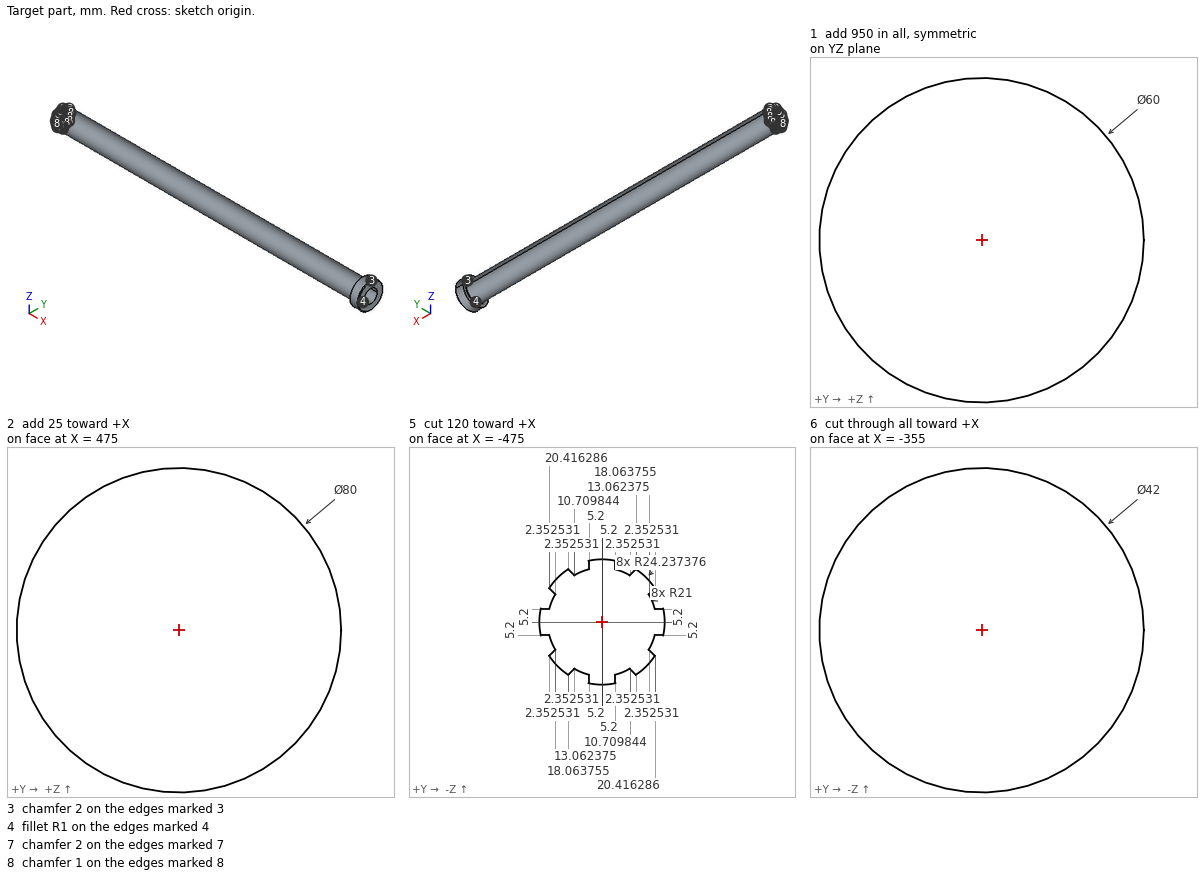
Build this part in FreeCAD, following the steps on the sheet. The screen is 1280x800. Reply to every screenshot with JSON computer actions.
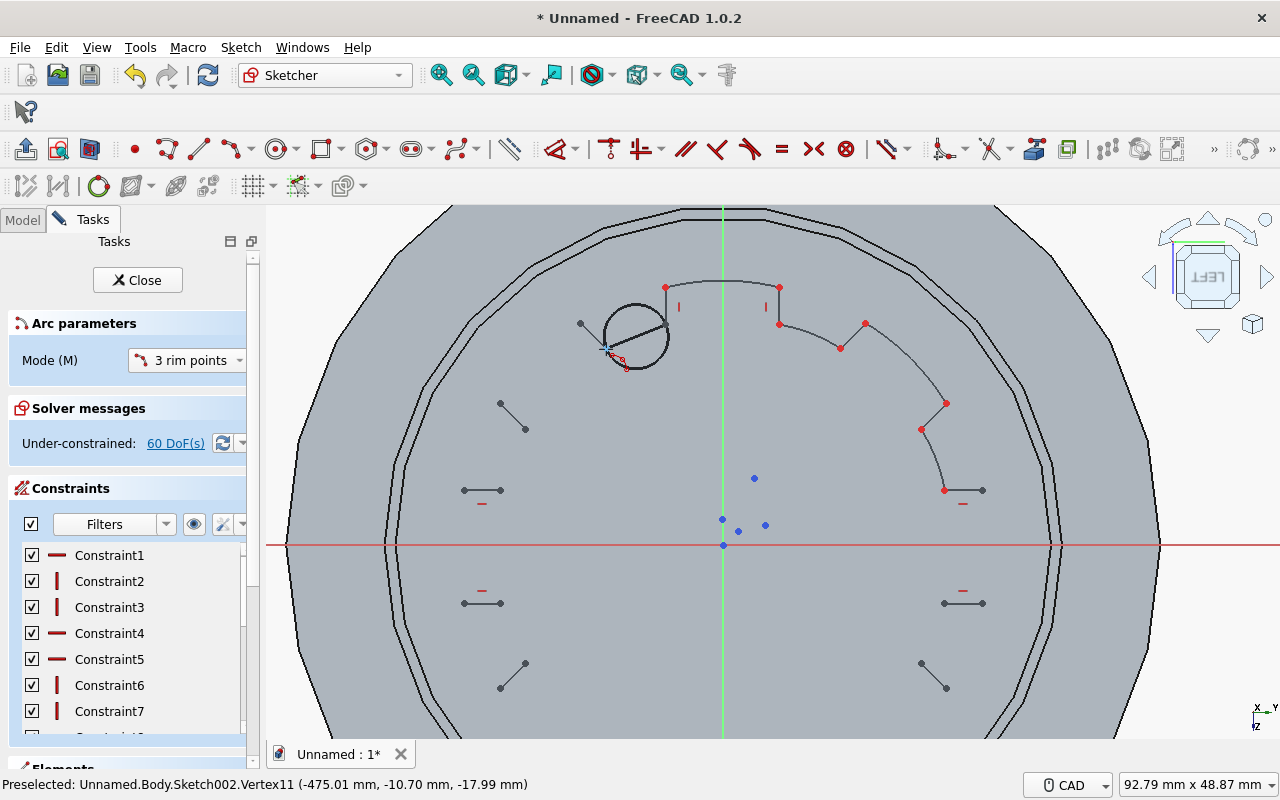
{"action": "scroll", "coordinate": [635, 333], "scroll_direction": "up", "scroll_amount": 10}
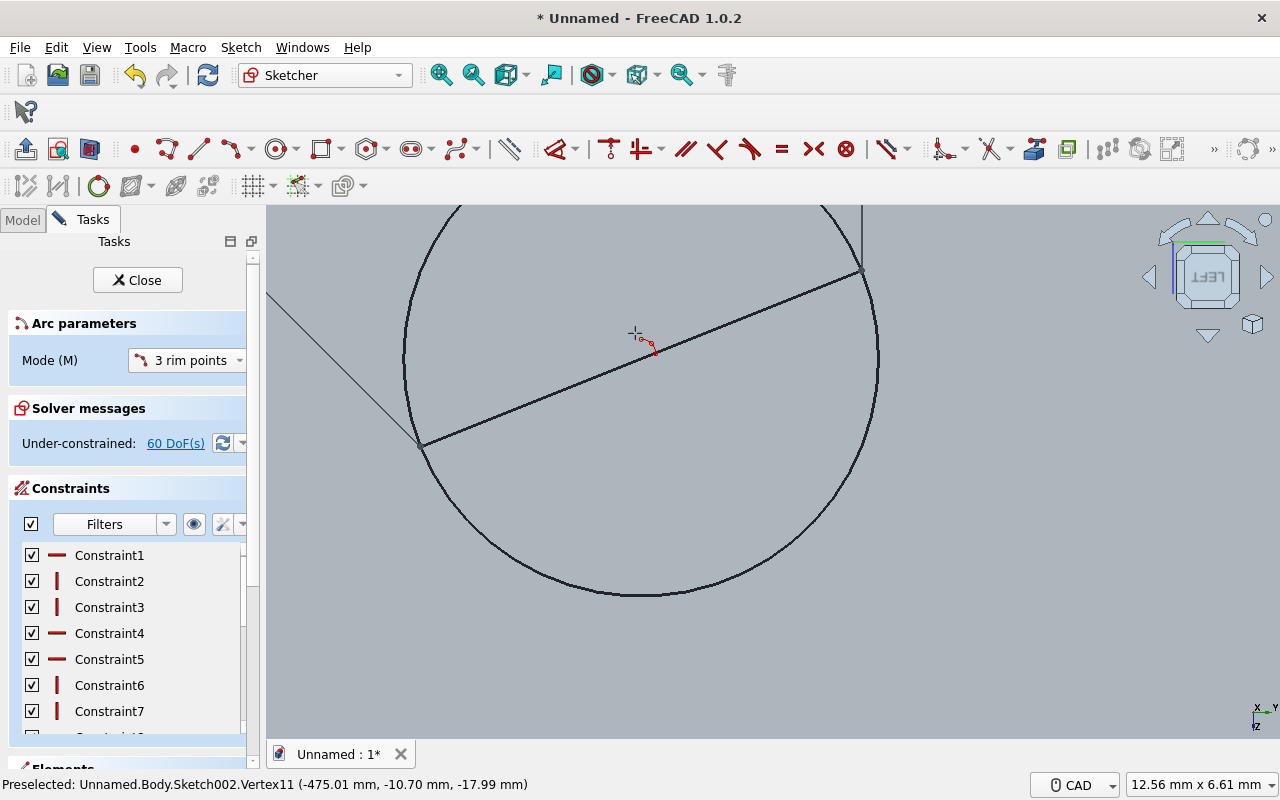
{"action": "left_click", "coordinate": [636, 333]}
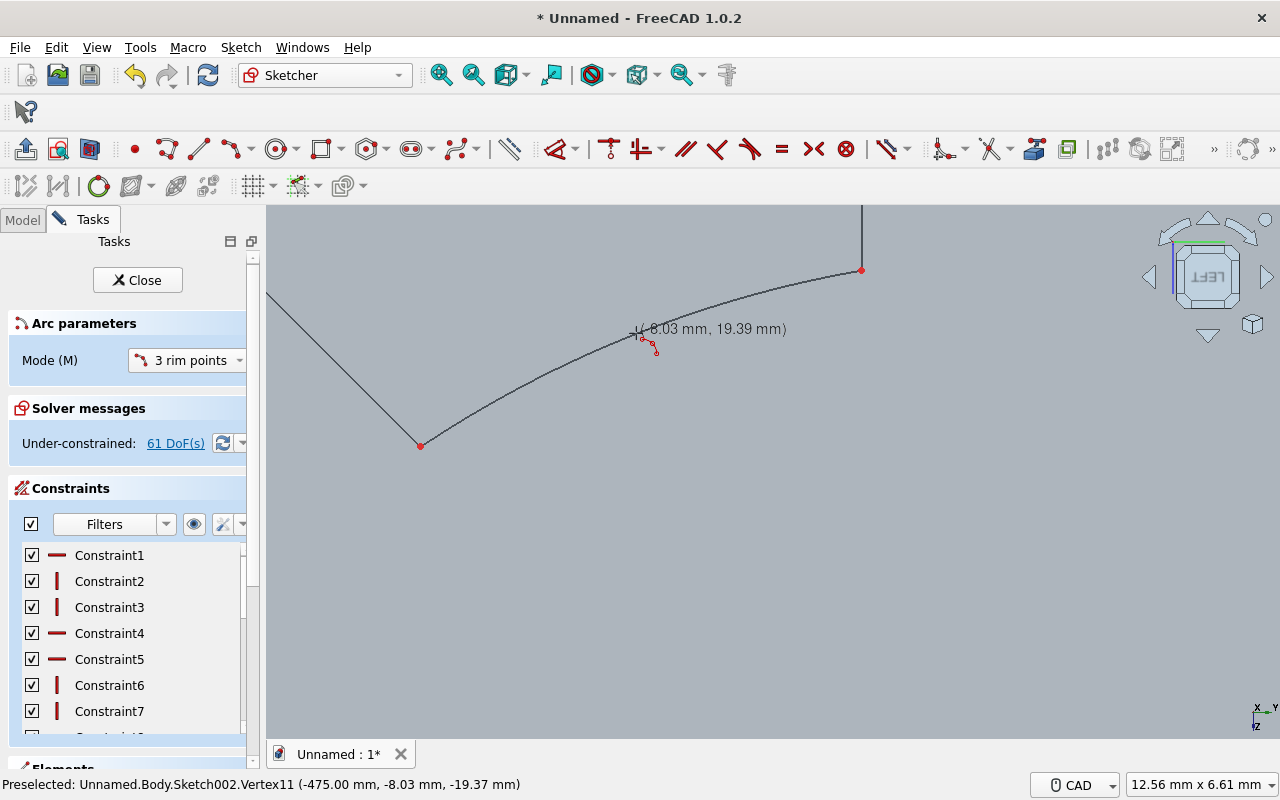
{"action": "scroll", "coordinate": [647, 330], "scroll_direction": "down", "scroll_amount": 12}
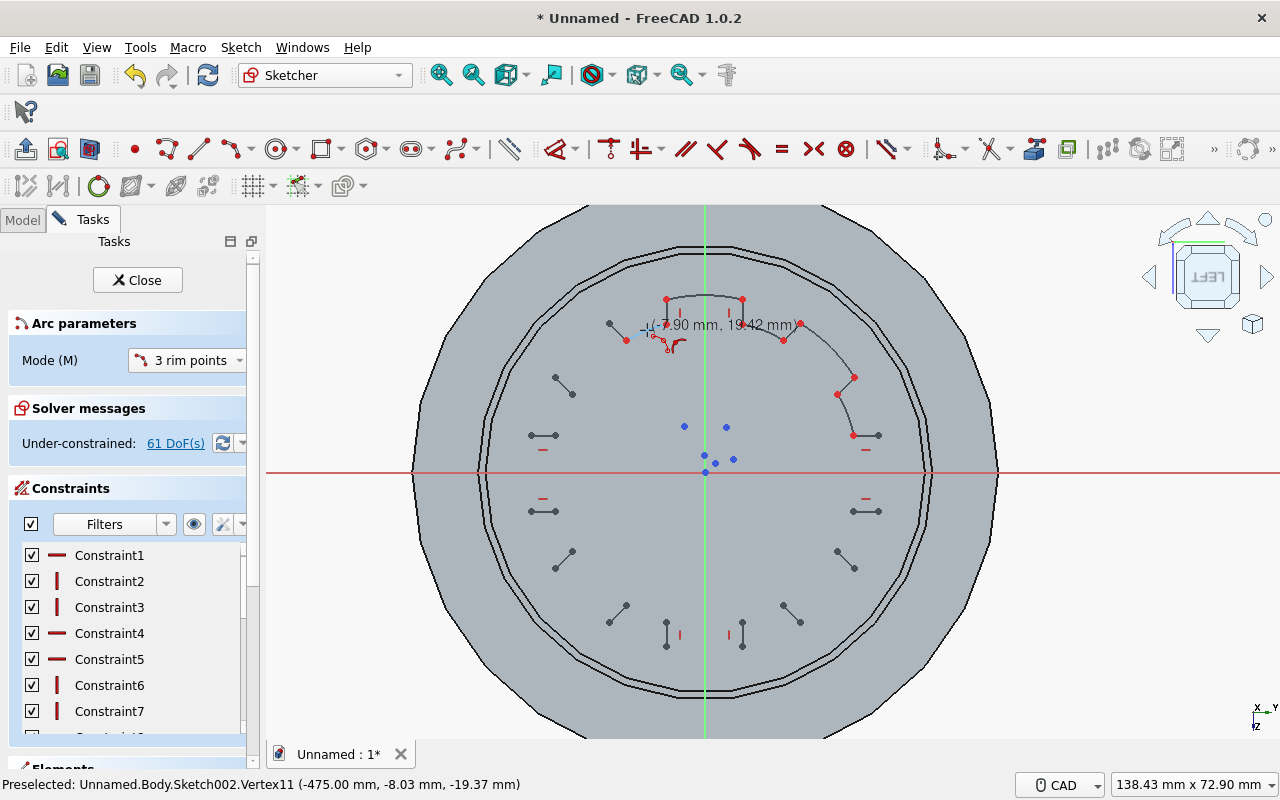
{"action": "scroll", "coordinate": [610, 323], "scroll_direction": "up", "scroll_amount": 2}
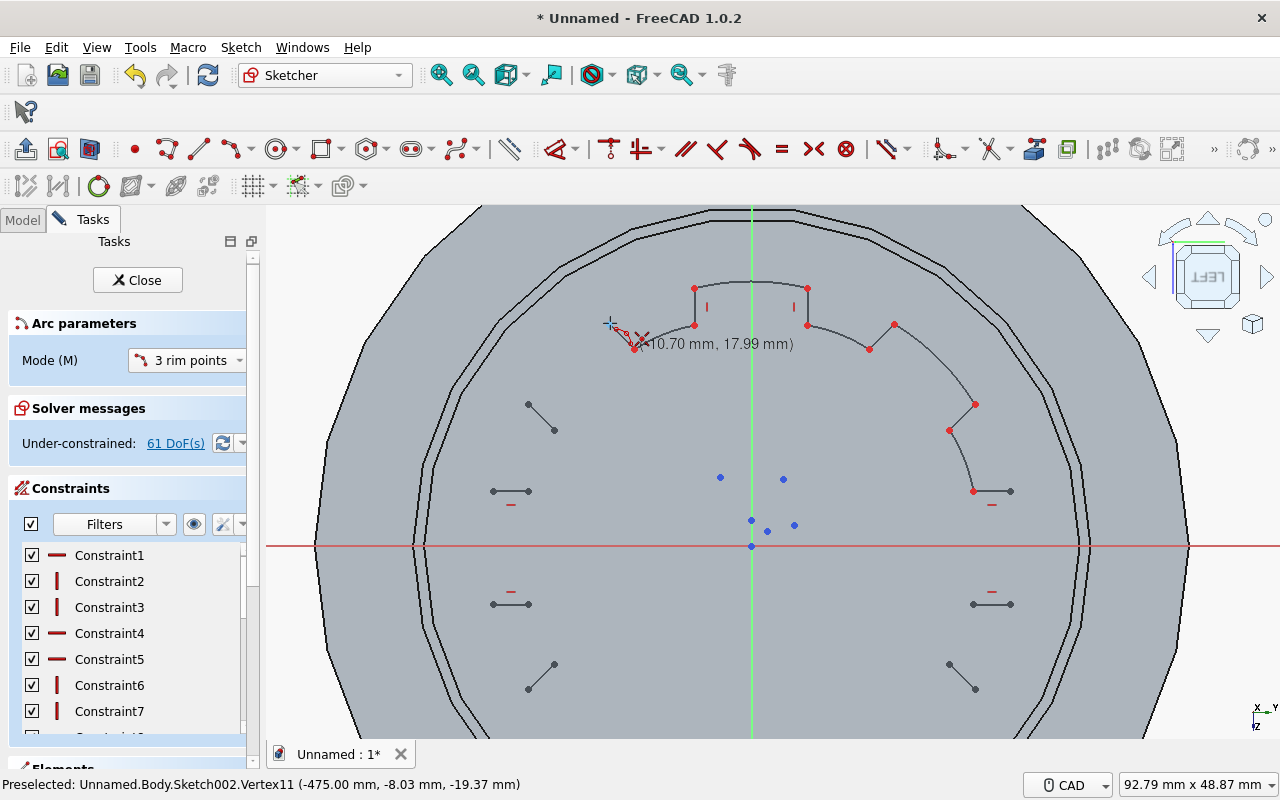
{"action": "left_click", "coordinate": [610, 324]}
{"action": "left_click", "coordinate": [529, 405]}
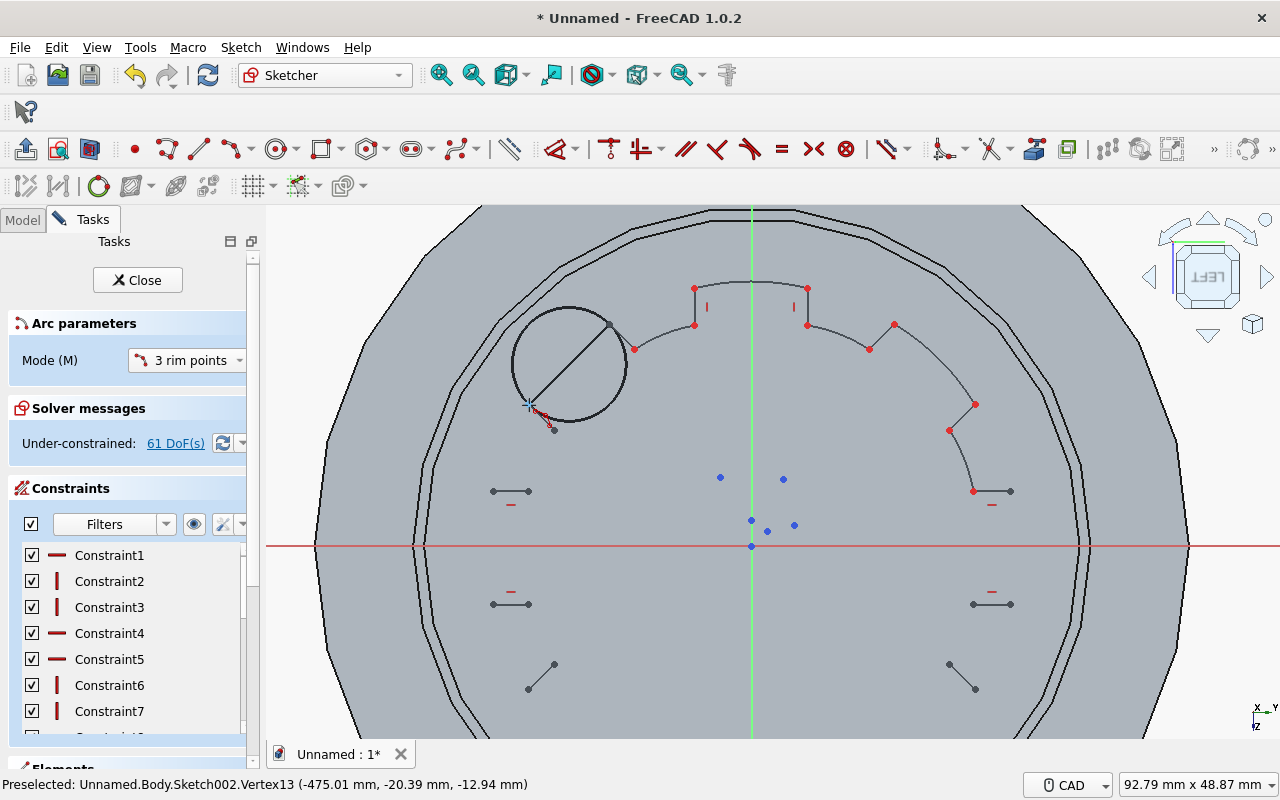
{"action": "scroll", "coordinate": [565, 359], "scroll_direction": "up", "scroll_amount": 5}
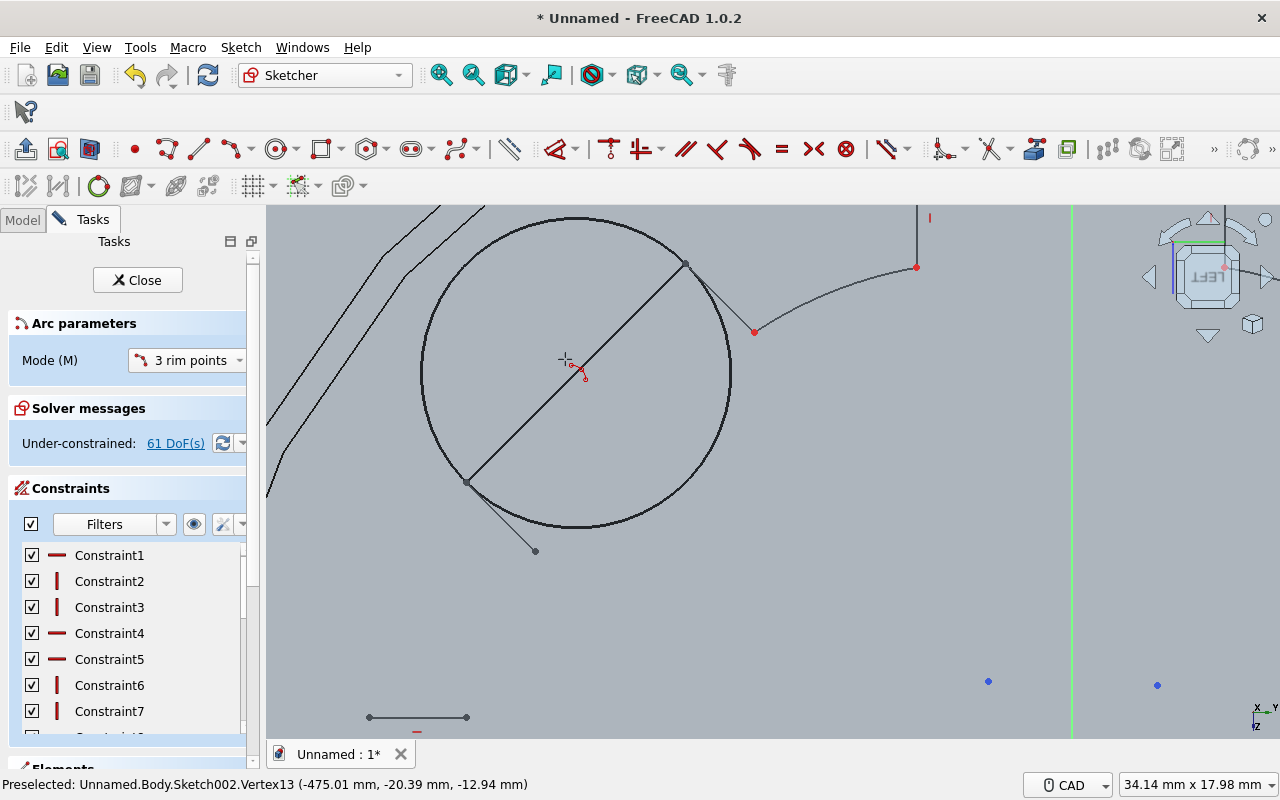
{"action": "left_click", "coordinate": [563, 358]}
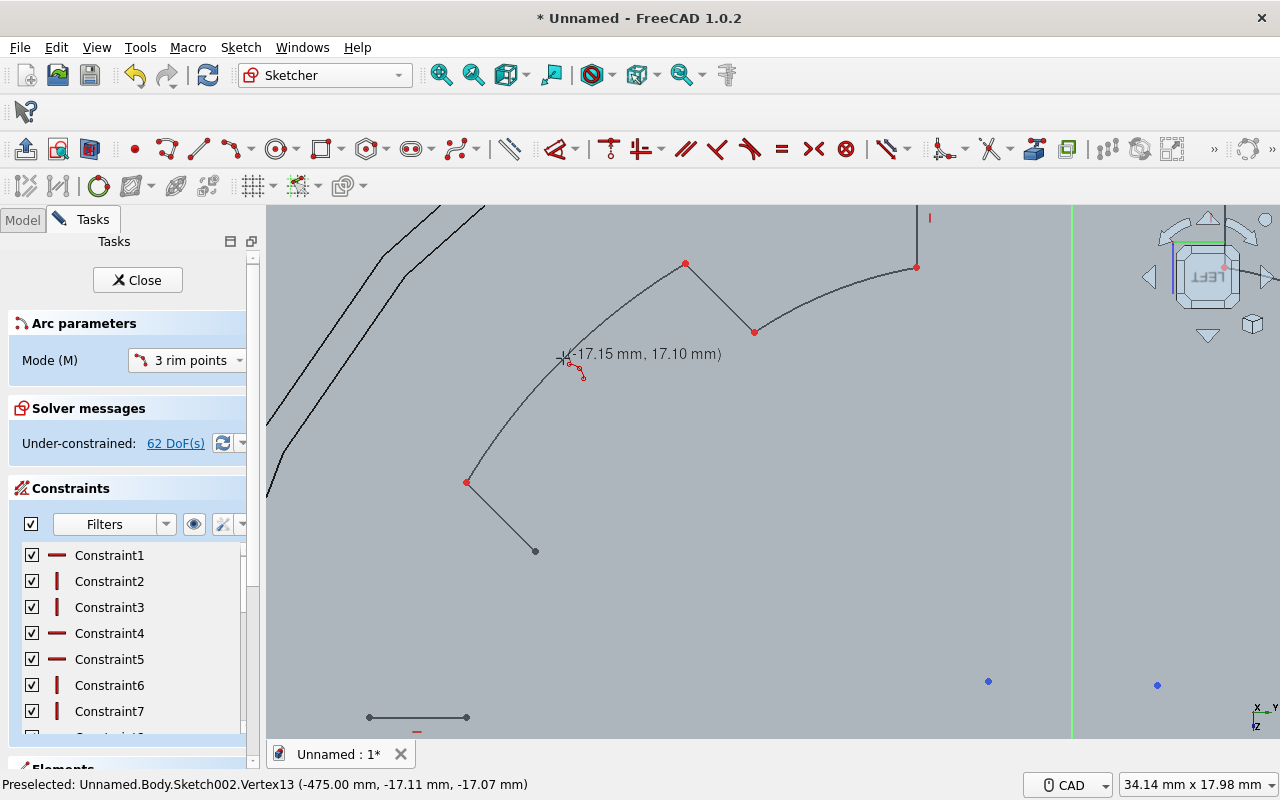
{"action": "scroll", "coordinate": [584, 343], "scroll_direction": "down", "scroll_amount": 7}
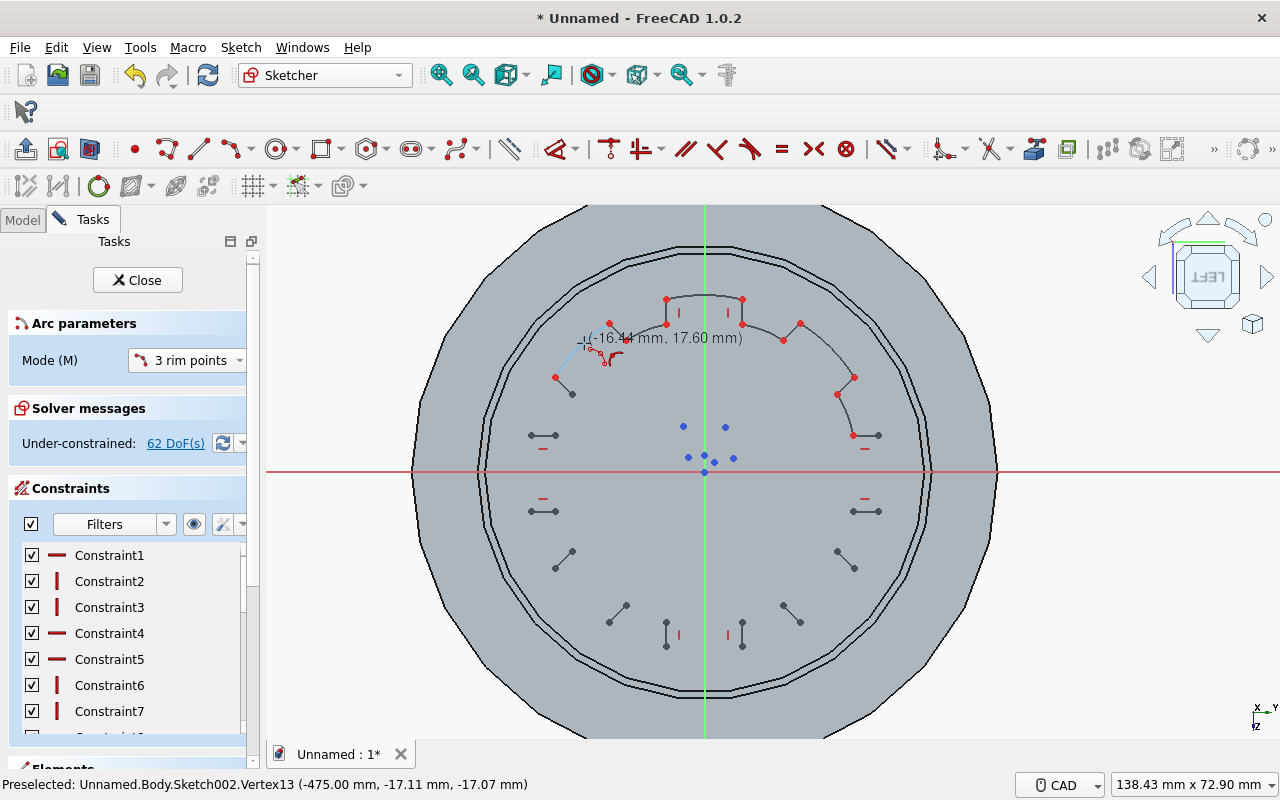
{"action": "scroll", "coordinate": [572, 394], "scroll_direction": "up", "scroll_amount": 2}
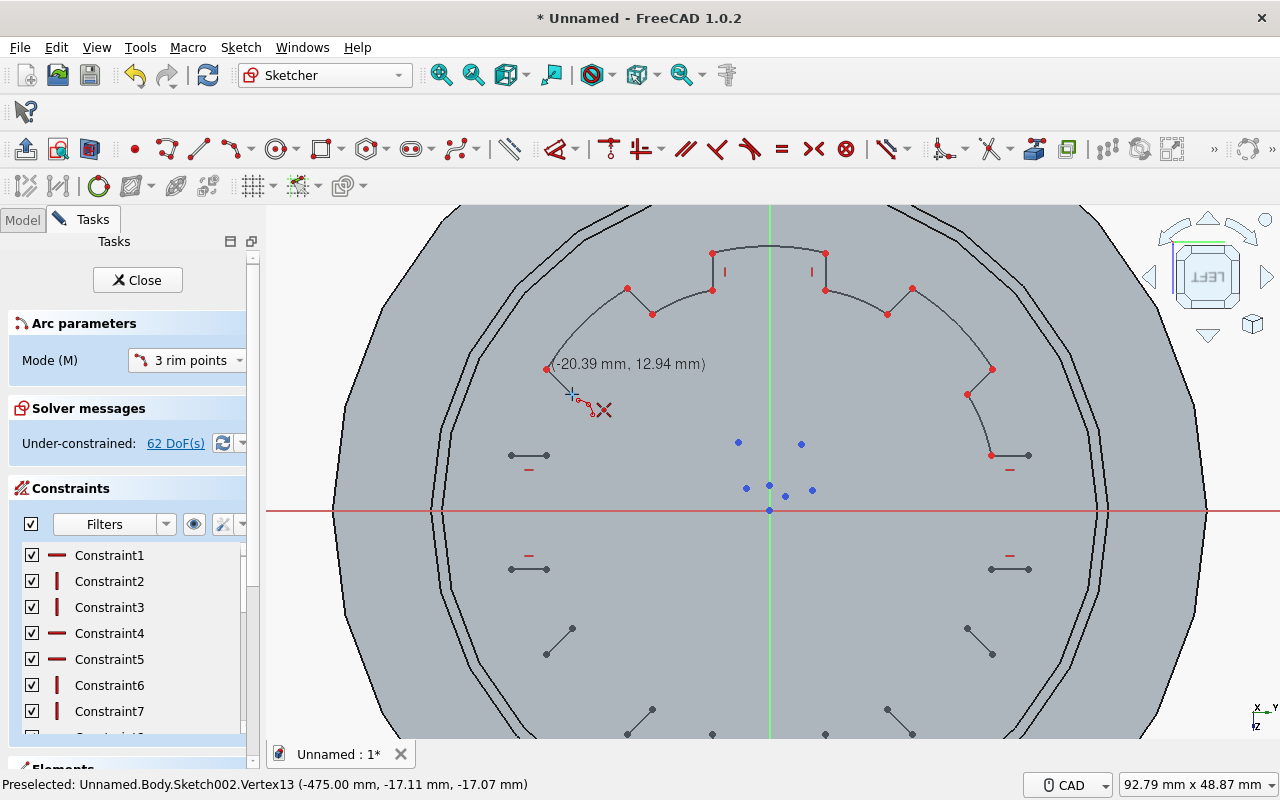
{"action": "left_click", "coordinate": [572, 395]}
{"action": "left_click", "coordinate": [547, 456]}